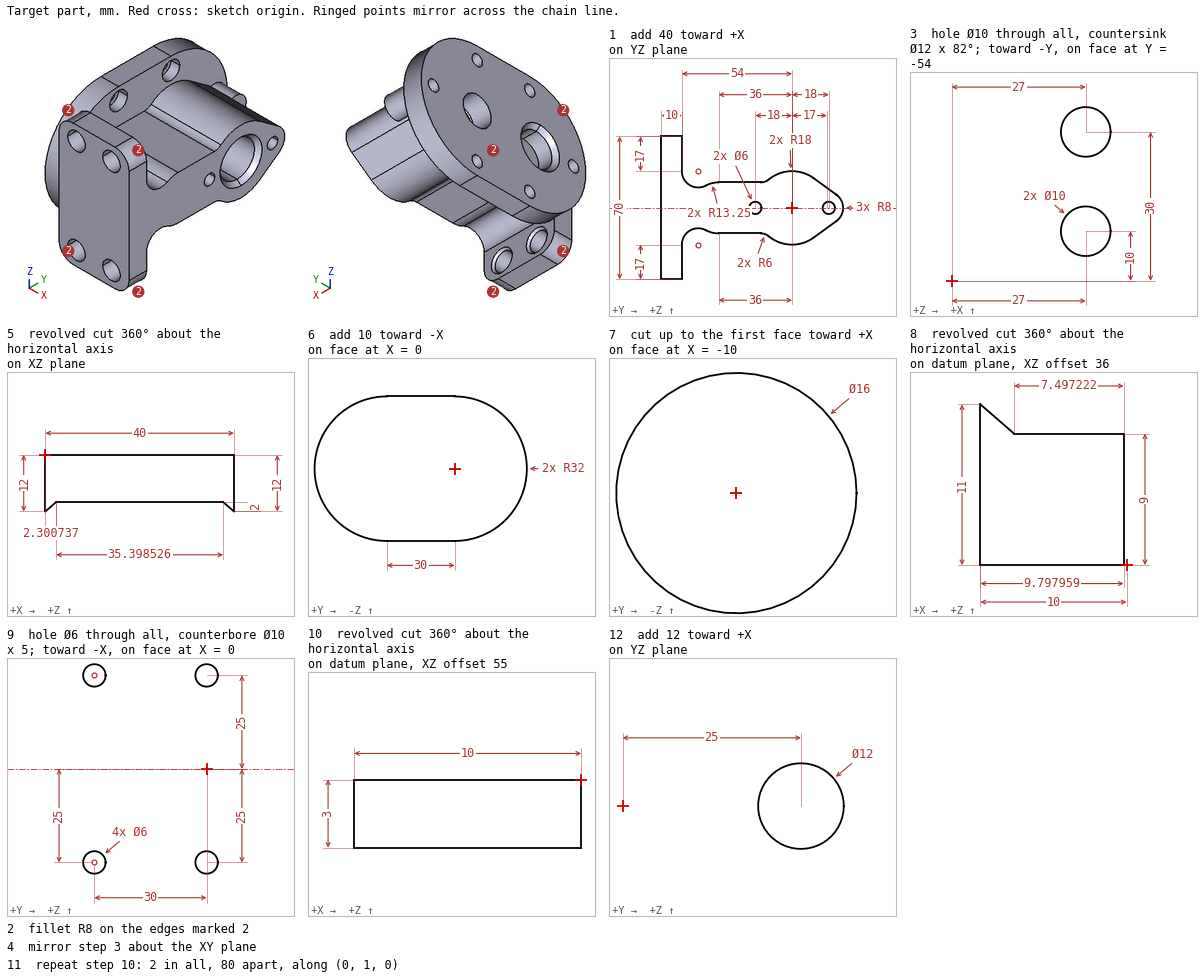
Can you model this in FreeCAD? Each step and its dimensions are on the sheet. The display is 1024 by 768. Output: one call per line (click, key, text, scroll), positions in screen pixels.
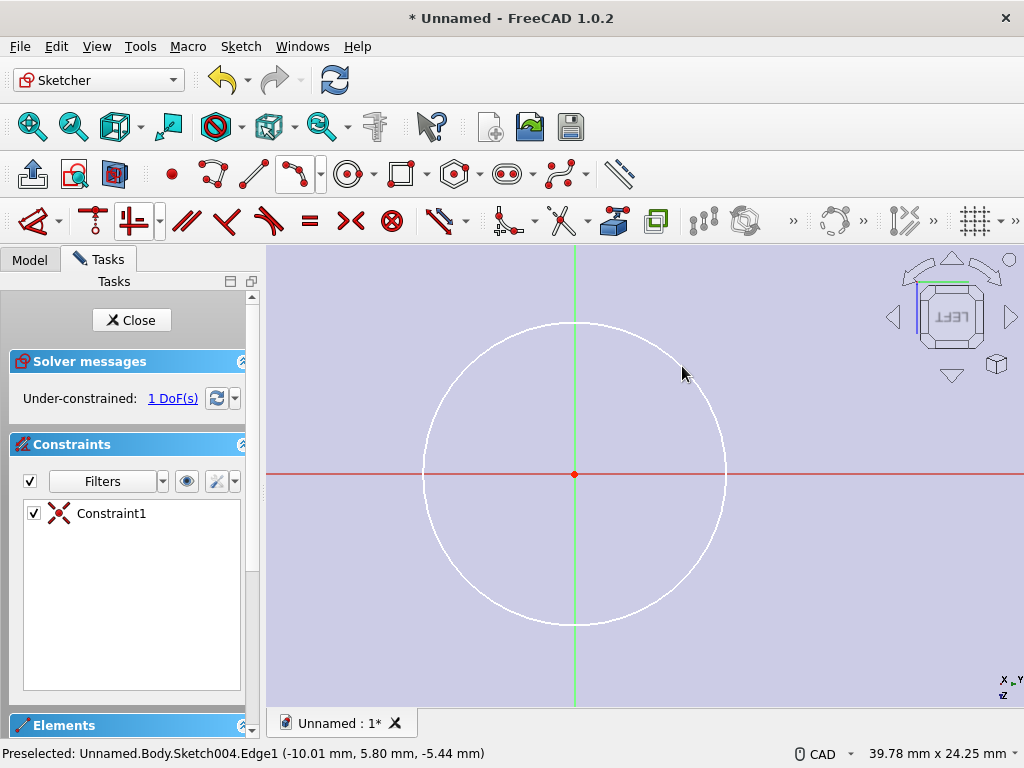
click(32, 222)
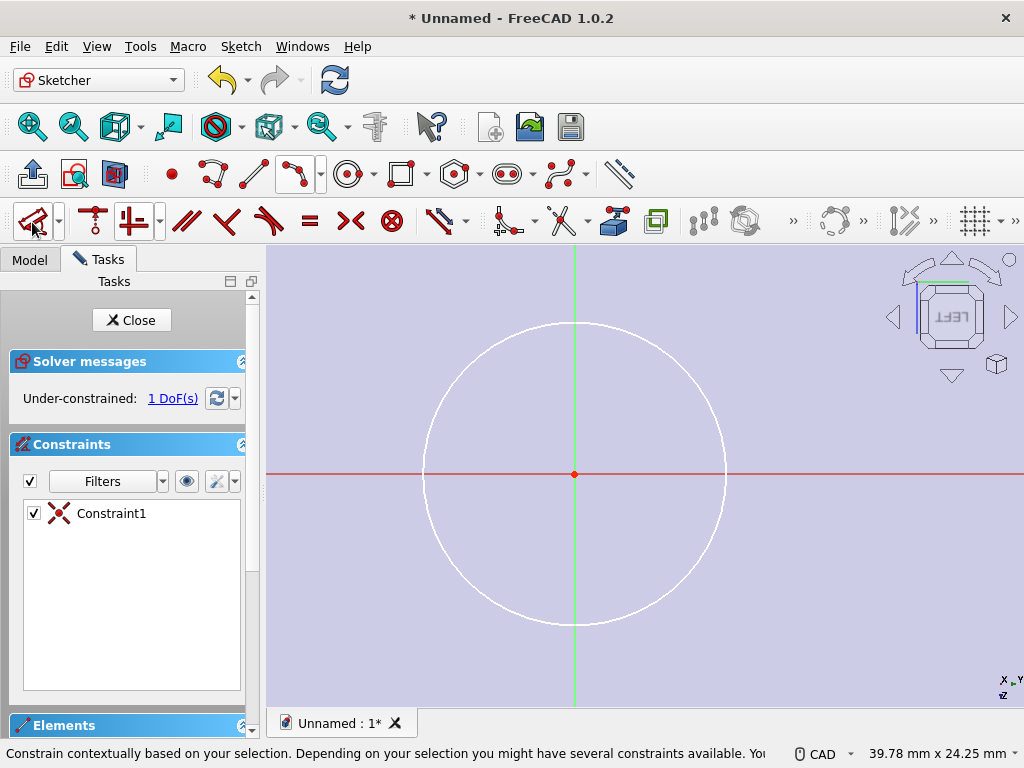
click(682, 367)
click(705, 344)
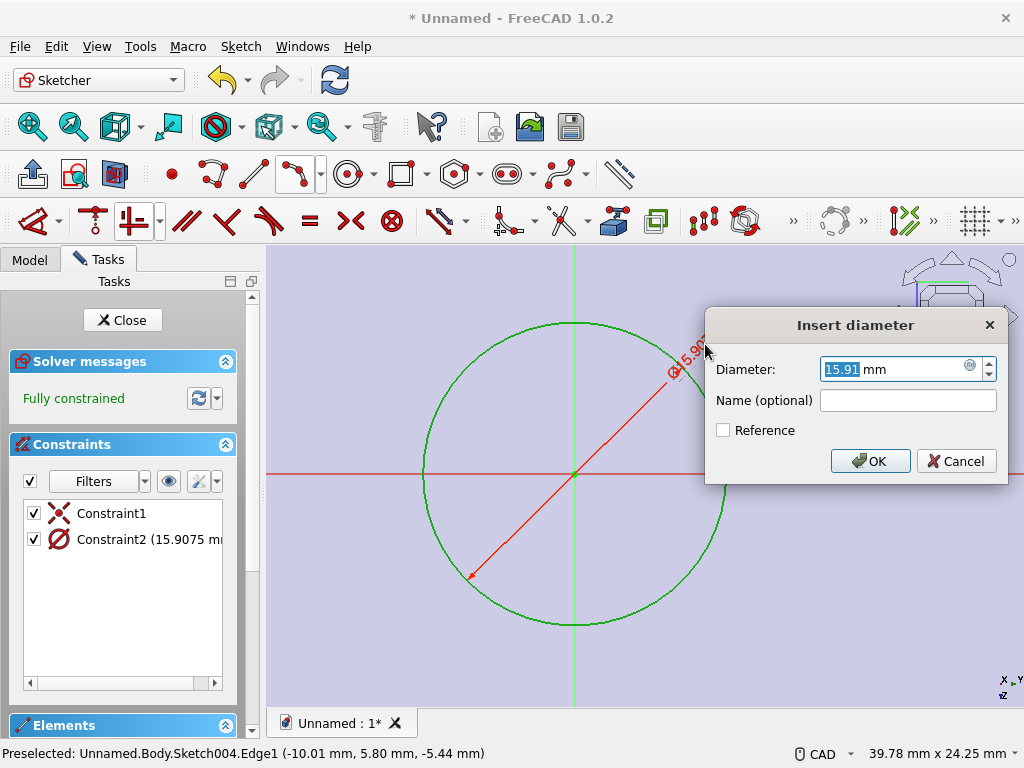
text(16)
key(Return)
key(Escape)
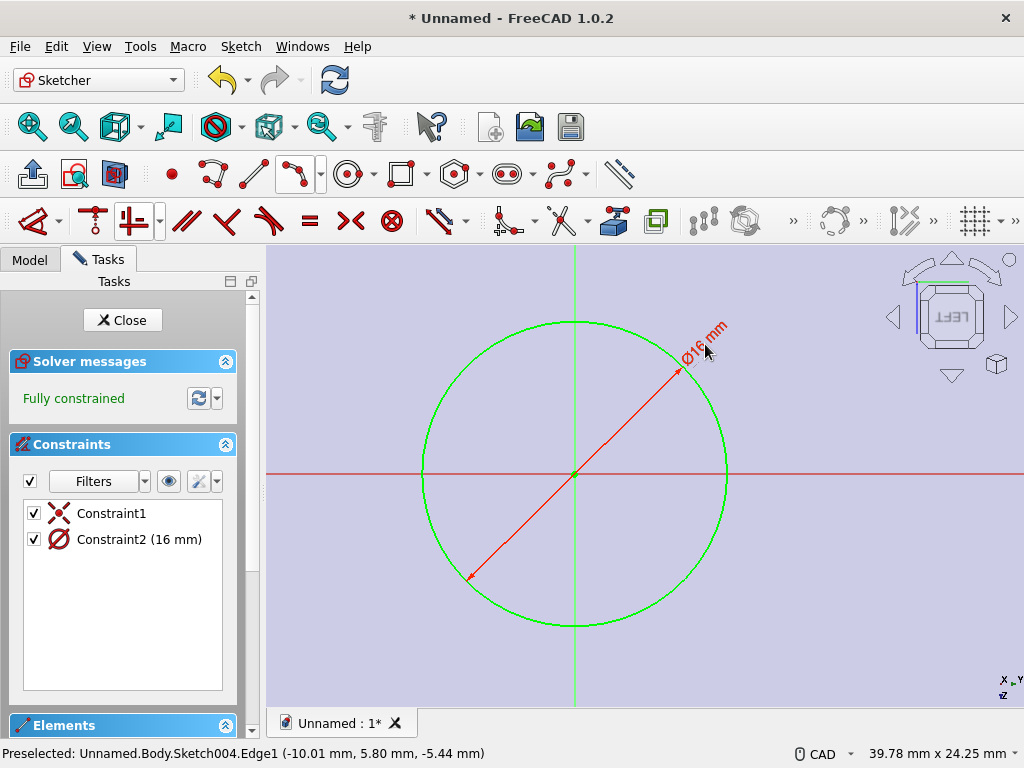
click(123, 320)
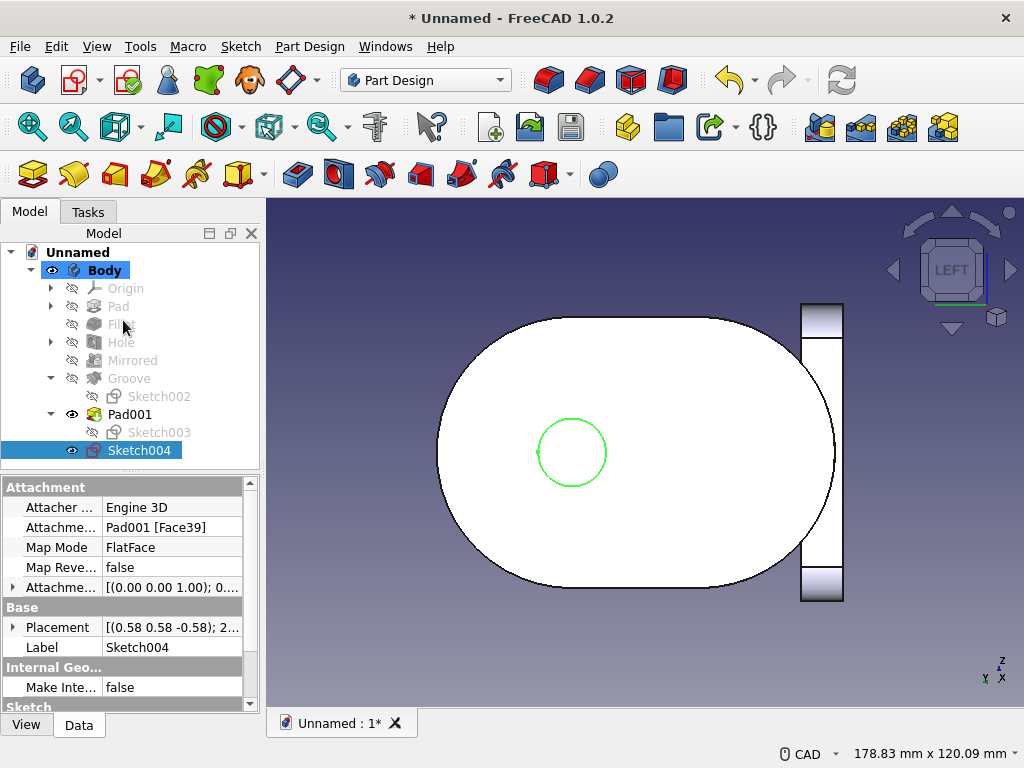
click(298, 174)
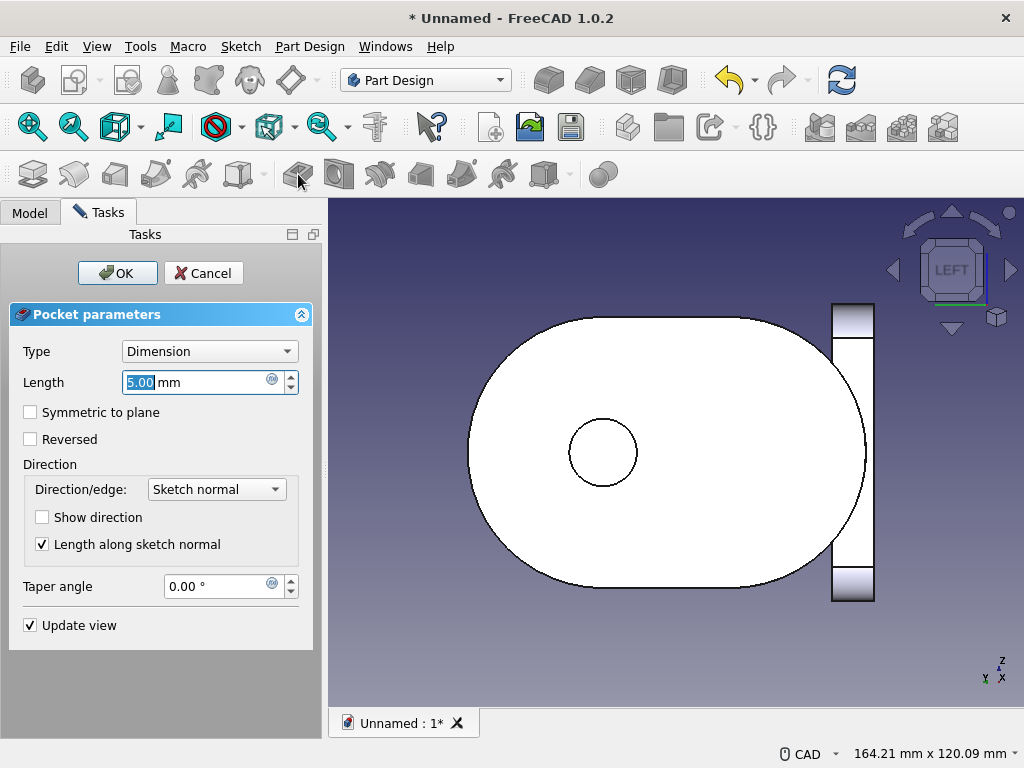
click(210, 352)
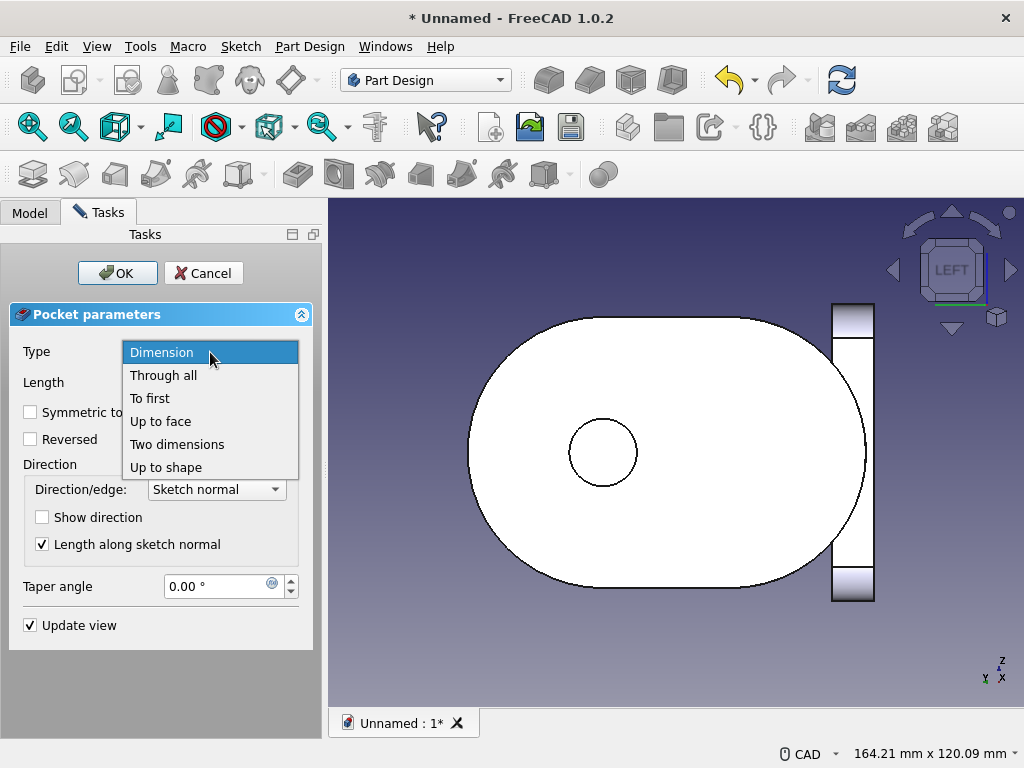
click(208, 398)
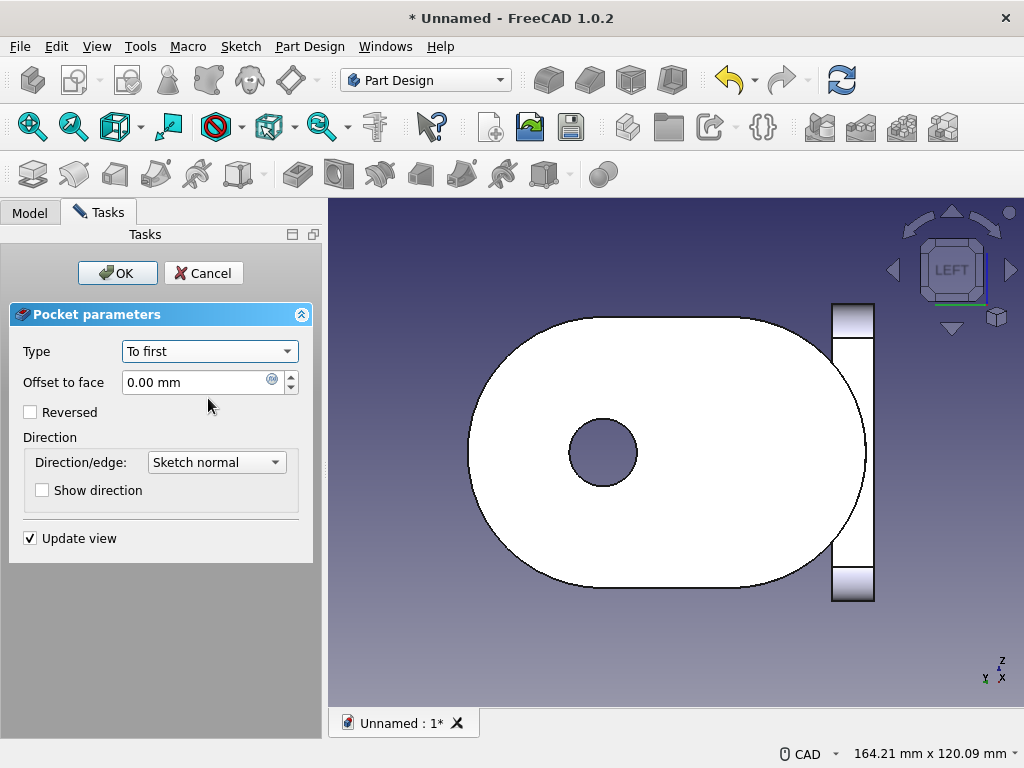
click(118, 273)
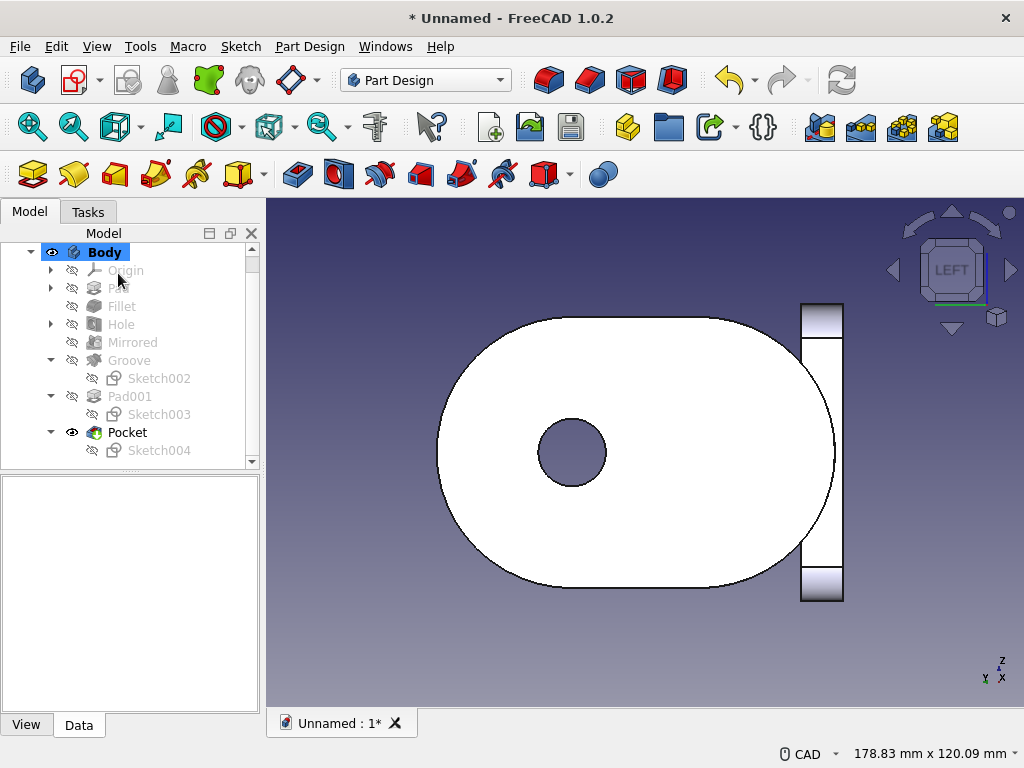
click(51, 270)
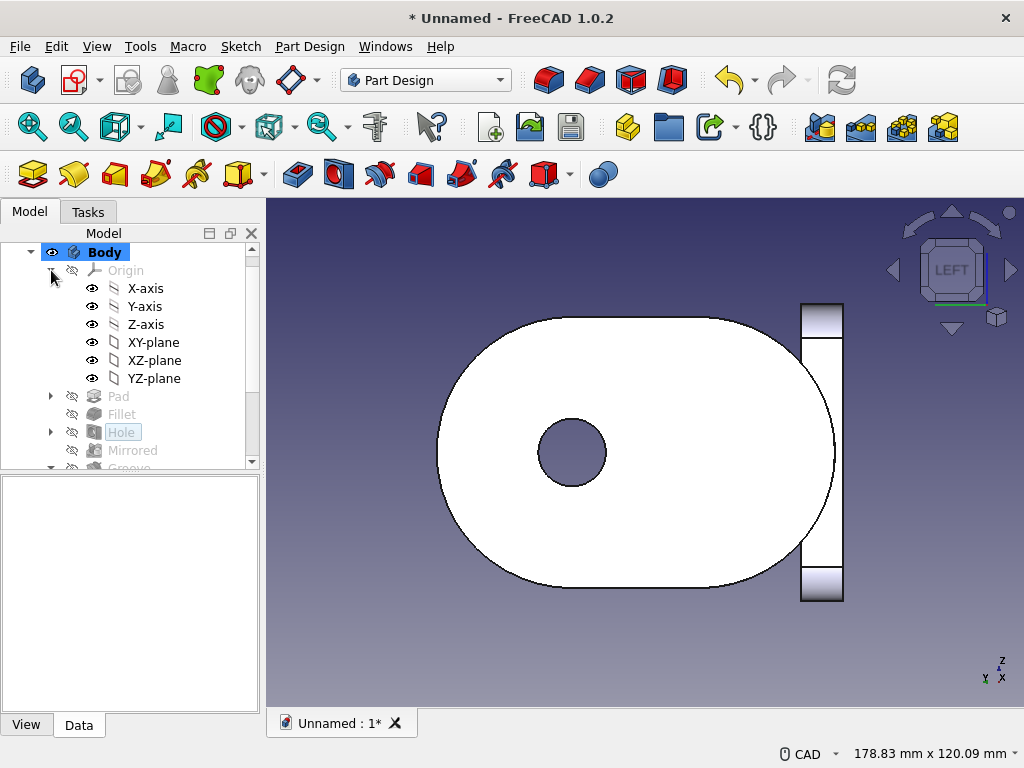
click(137, 360)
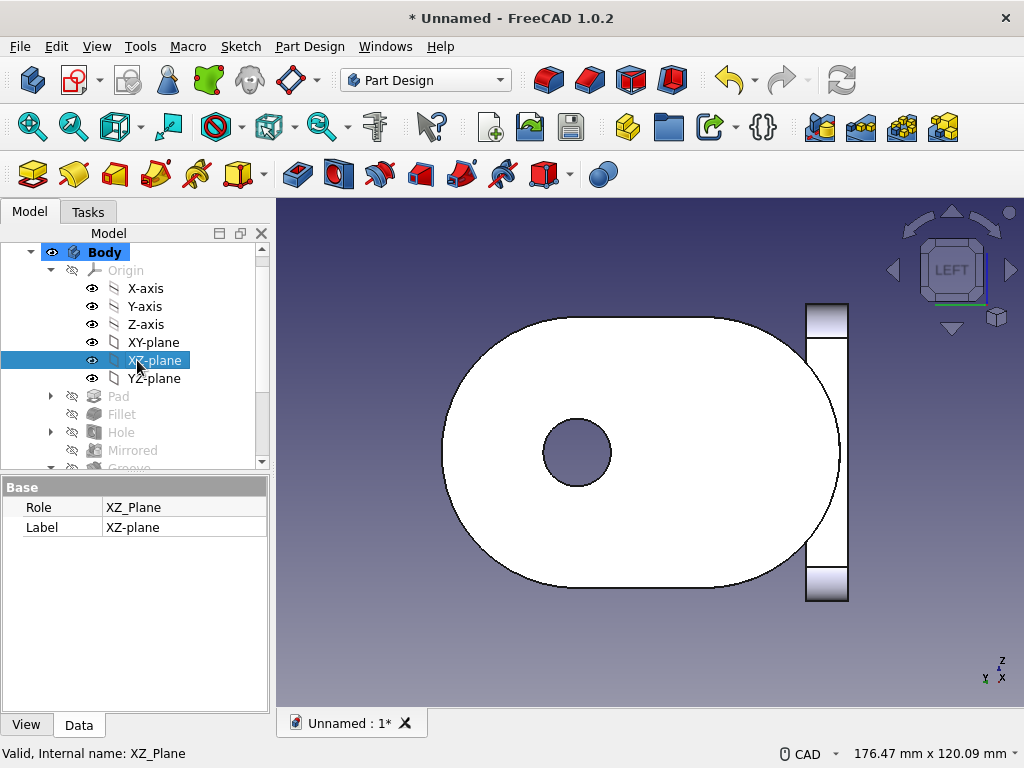
click(290, 80)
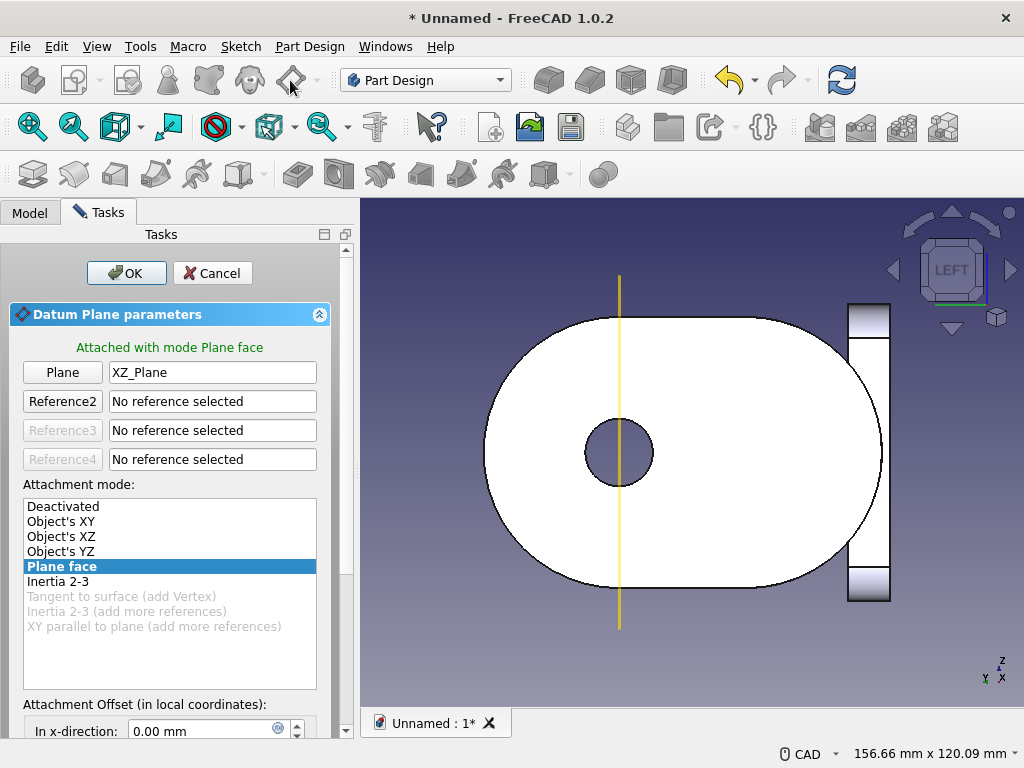
scroll(346, 491, down, 3)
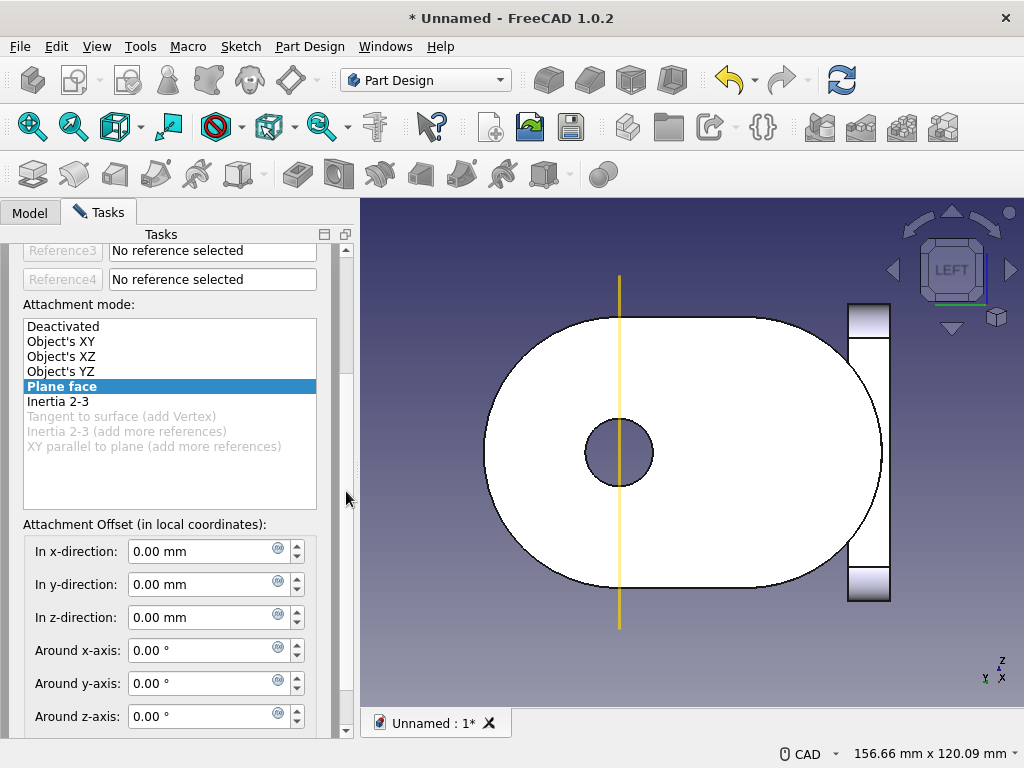
triple_click(210, 618)